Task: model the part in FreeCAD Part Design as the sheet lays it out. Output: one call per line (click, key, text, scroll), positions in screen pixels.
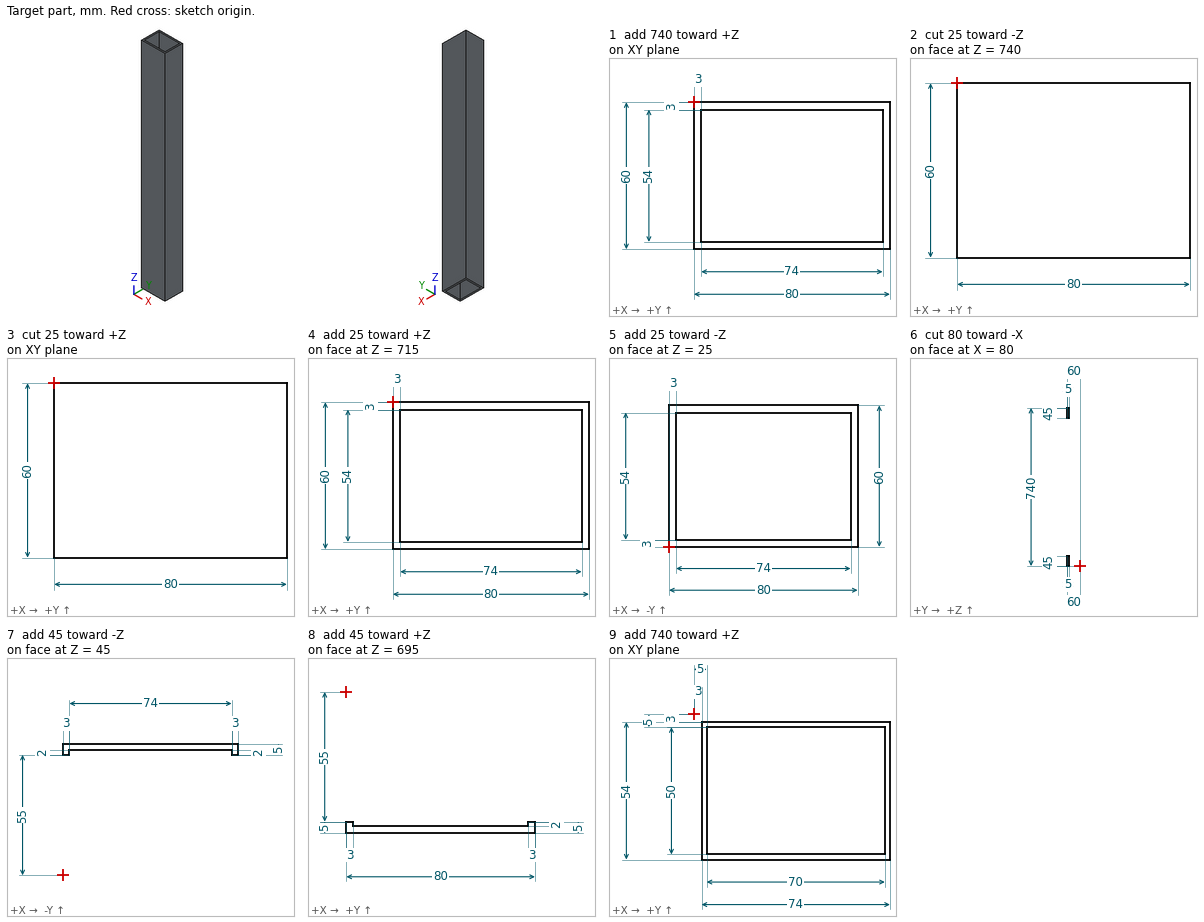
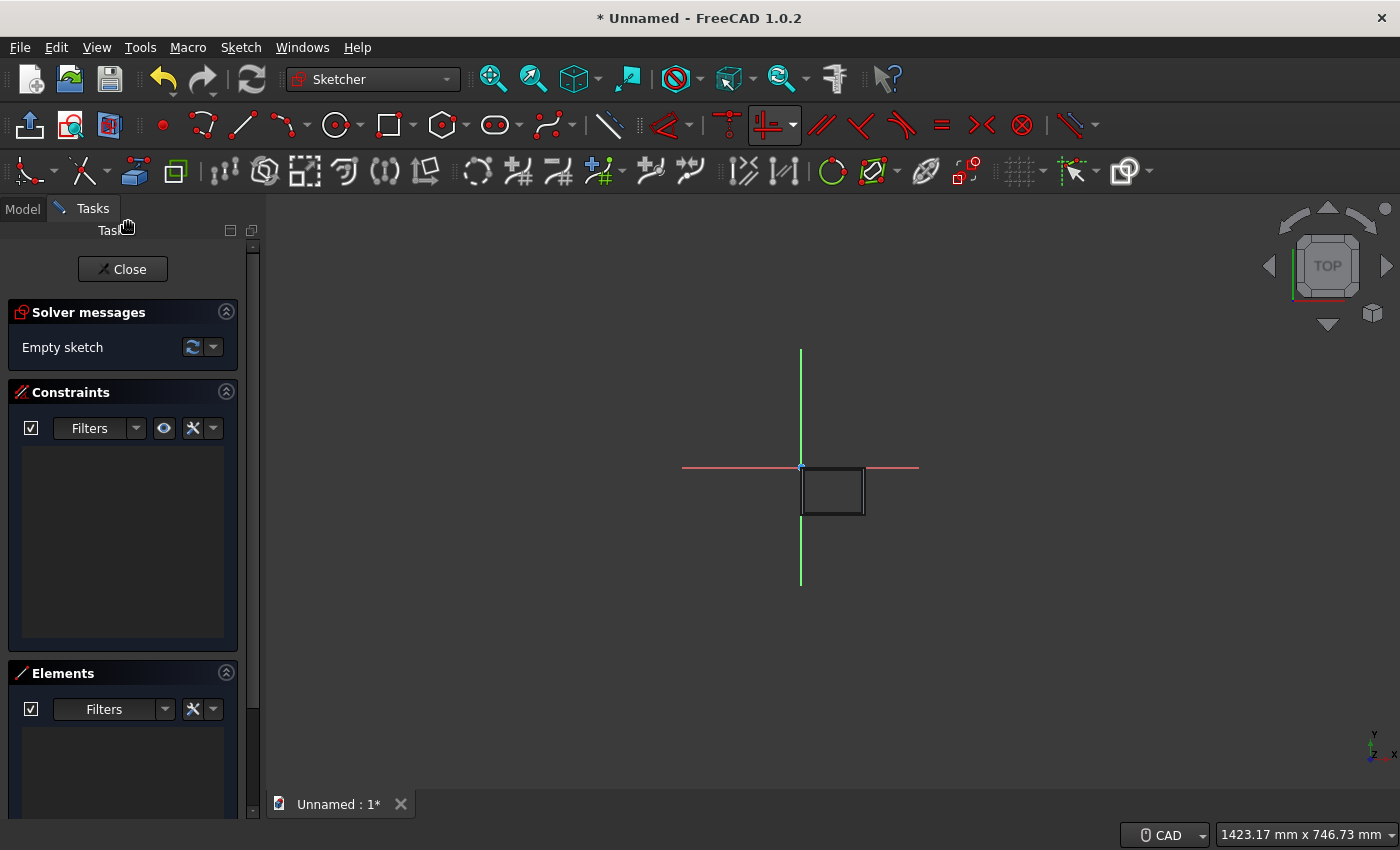
click(110, 126)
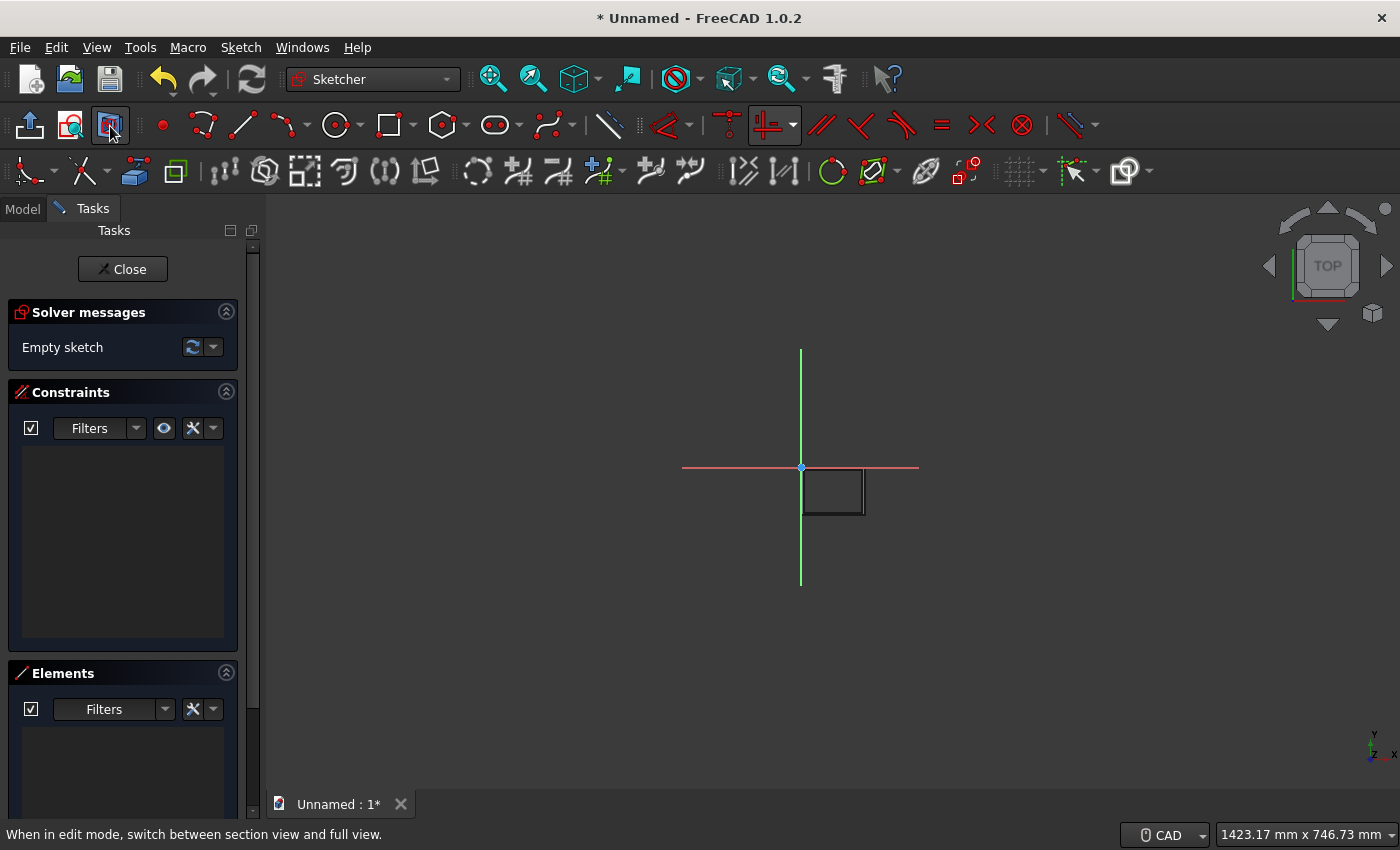
scroll(840, 490, up, 11)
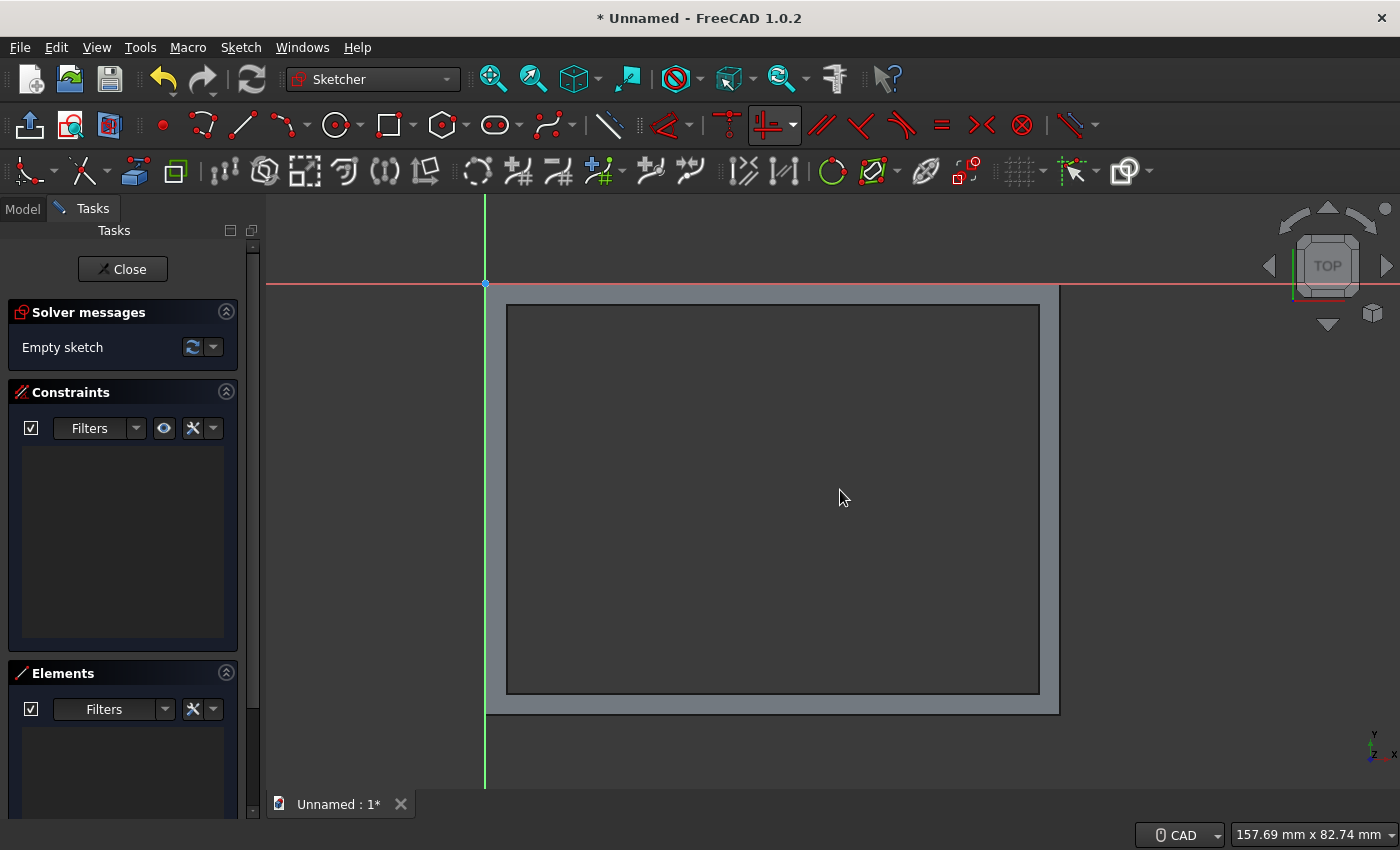
key(g)
key(r)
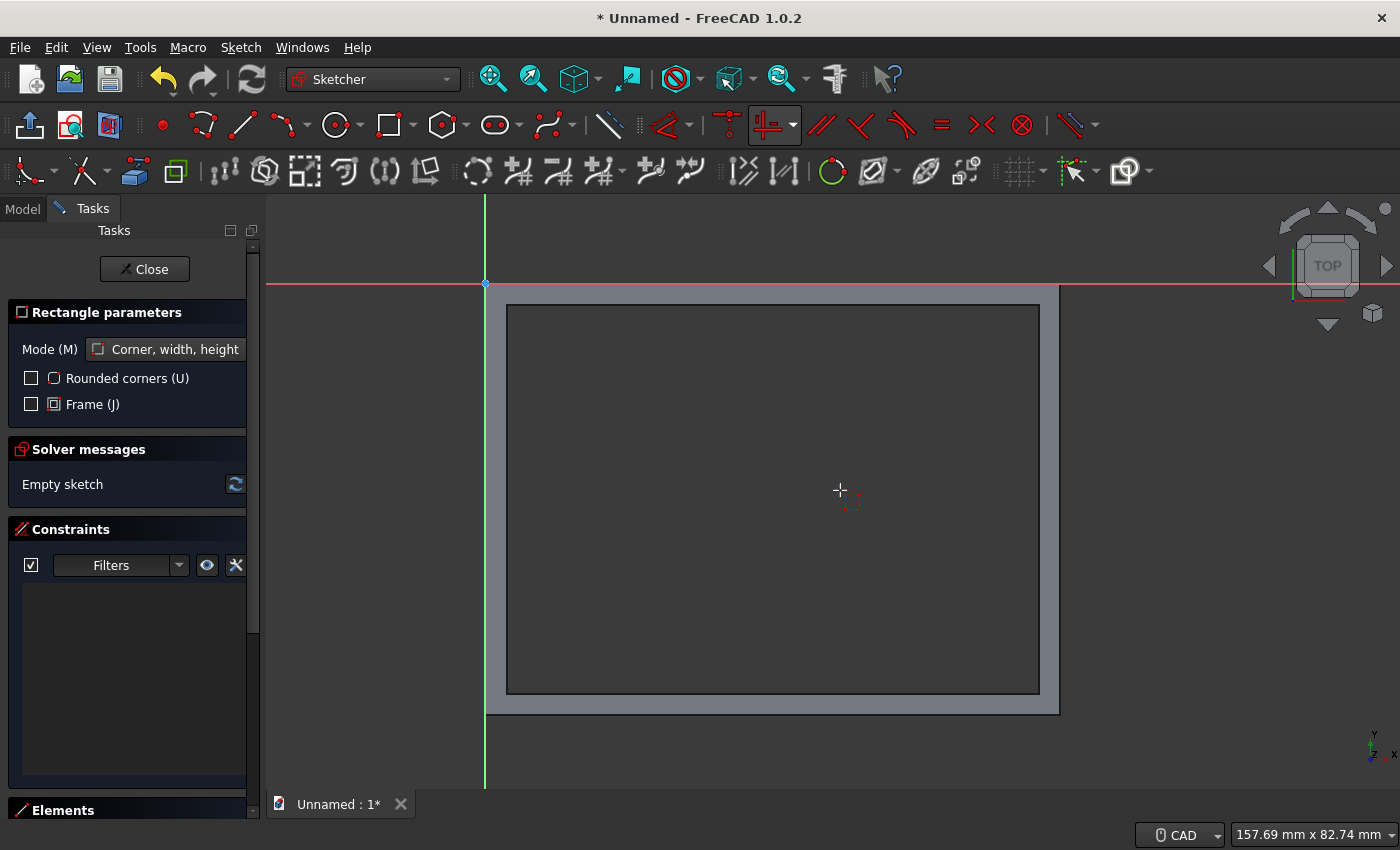
click(507, 305)
click(1039, 694)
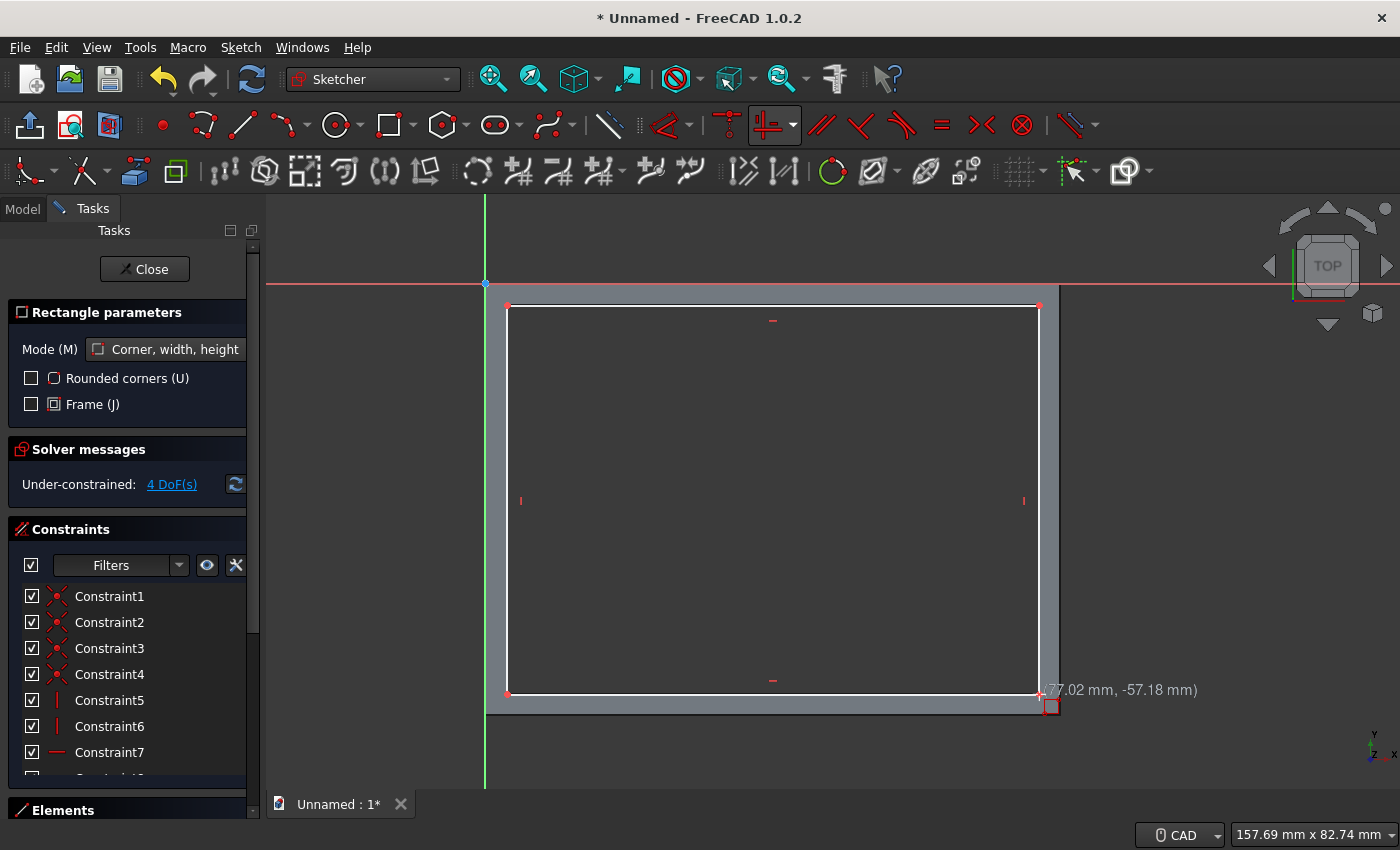
click(521, 320)
click(1024, 679)
key(Escape)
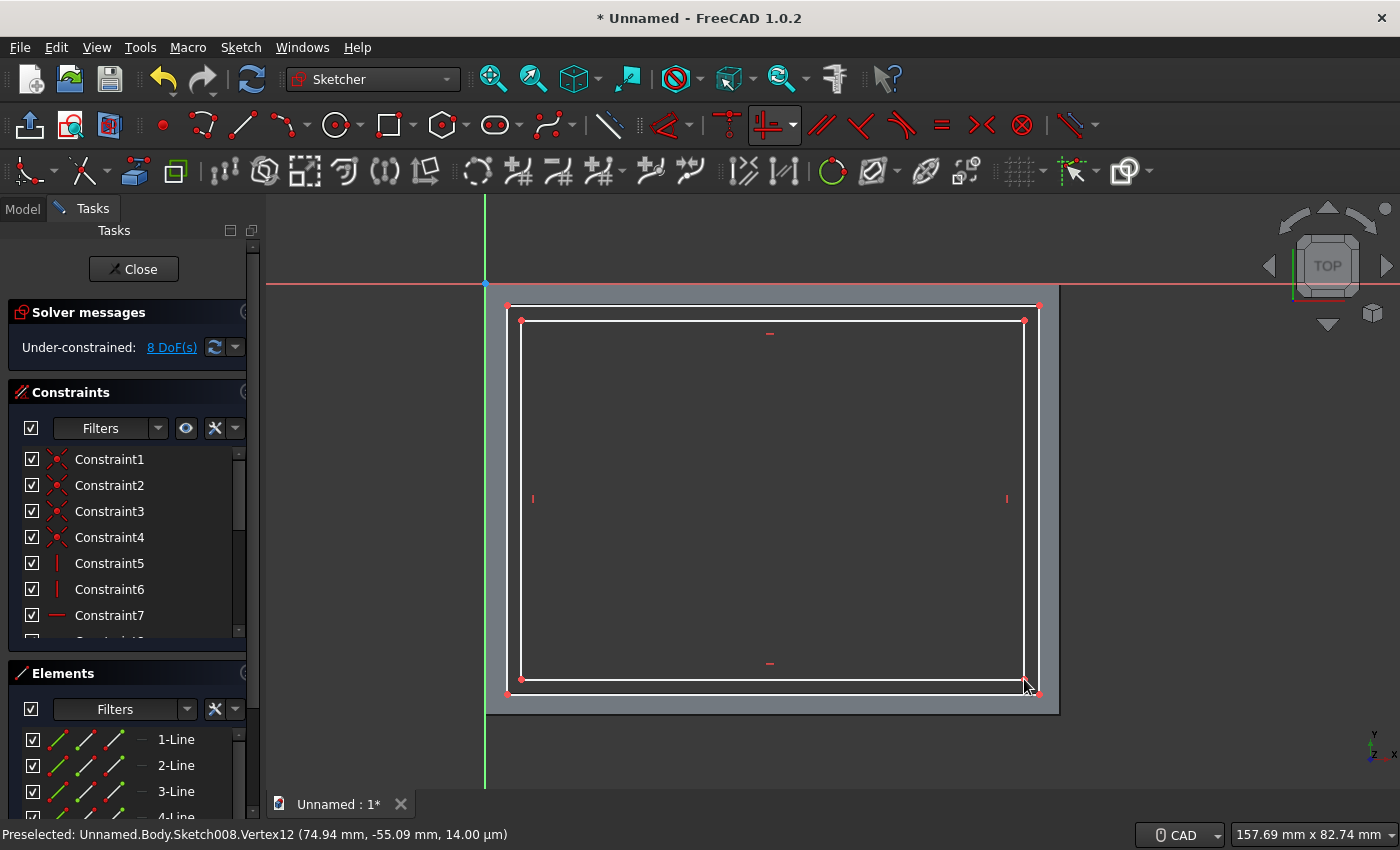
key(d)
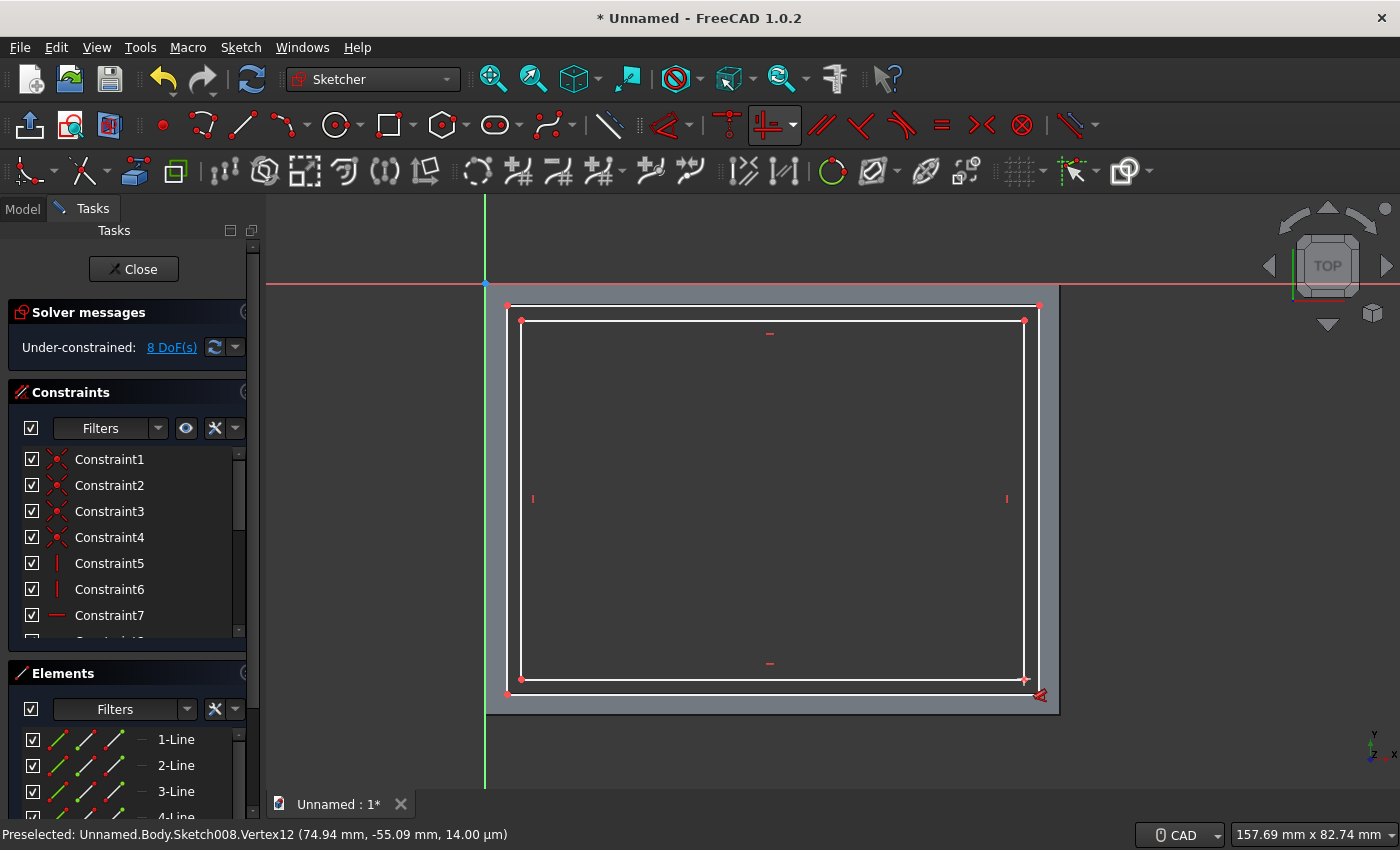
click(507, 423)
click(541, 500)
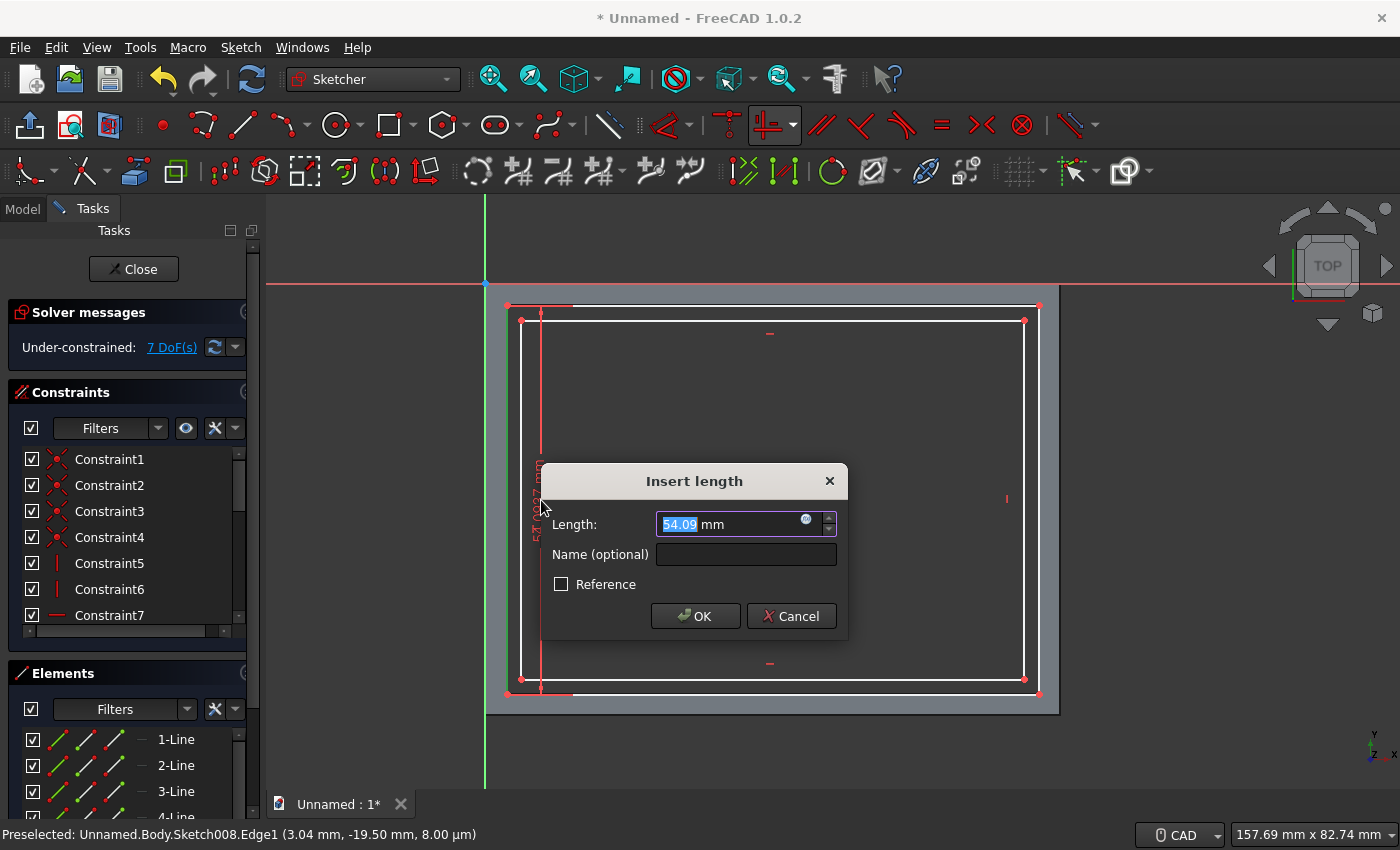
text(54)
key(Return)